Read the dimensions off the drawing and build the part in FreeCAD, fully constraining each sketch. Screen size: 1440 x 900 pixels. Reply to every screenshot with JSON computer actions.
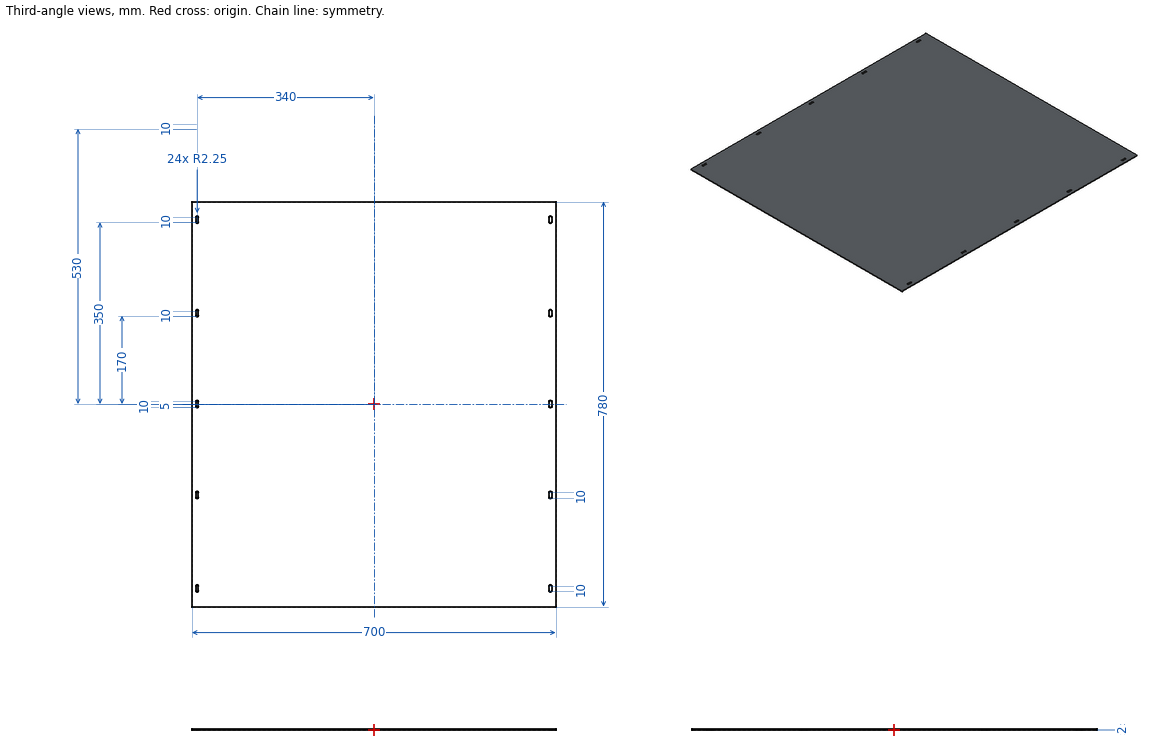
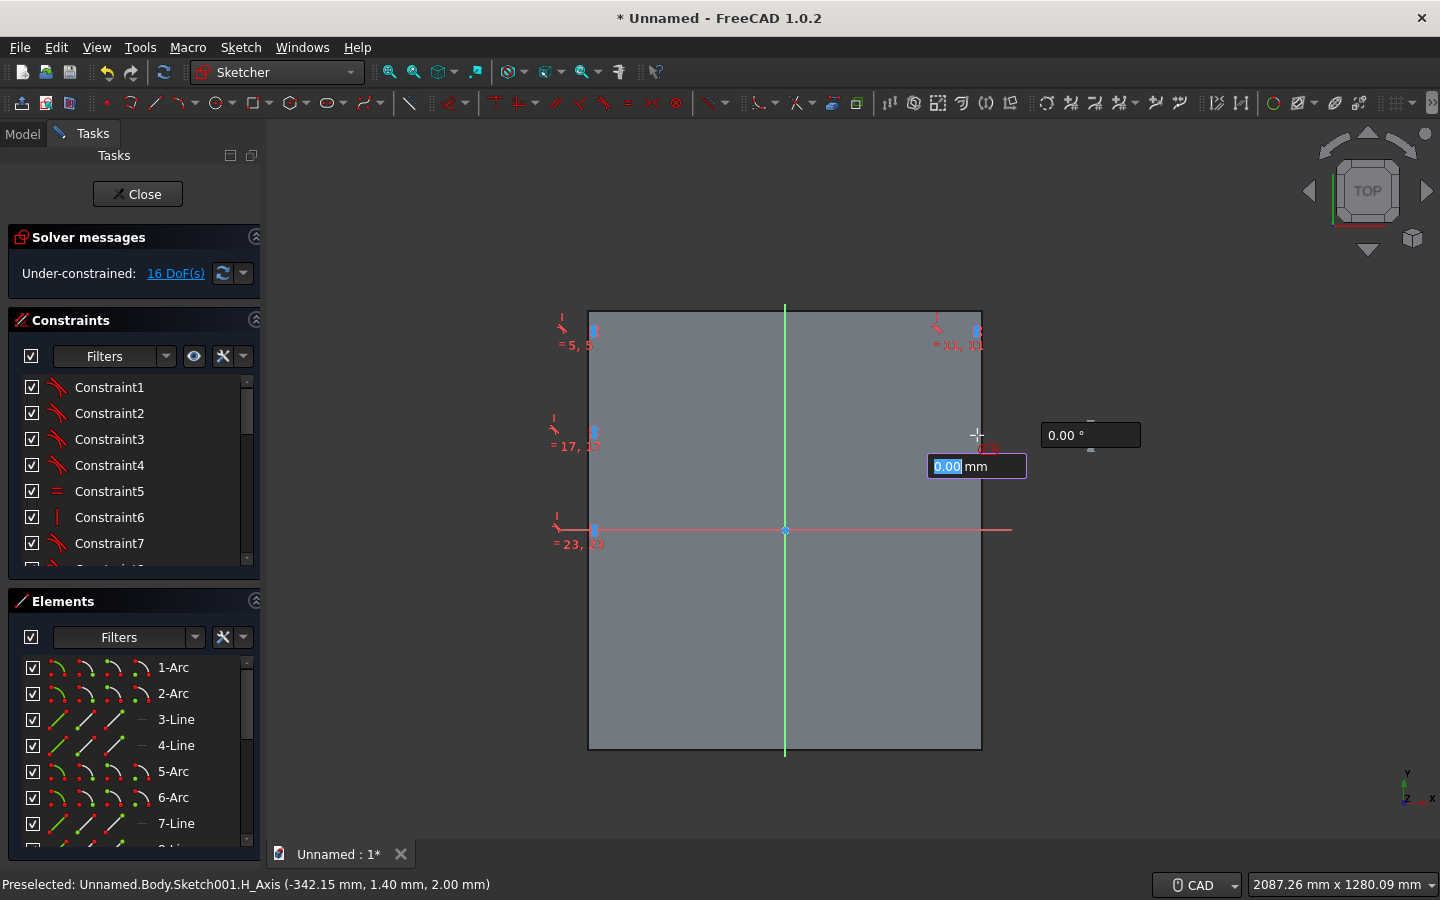
{"action": "scroll", "coordinate": [977, 429], "scroll_direction": "up", "scroll_amount": 6}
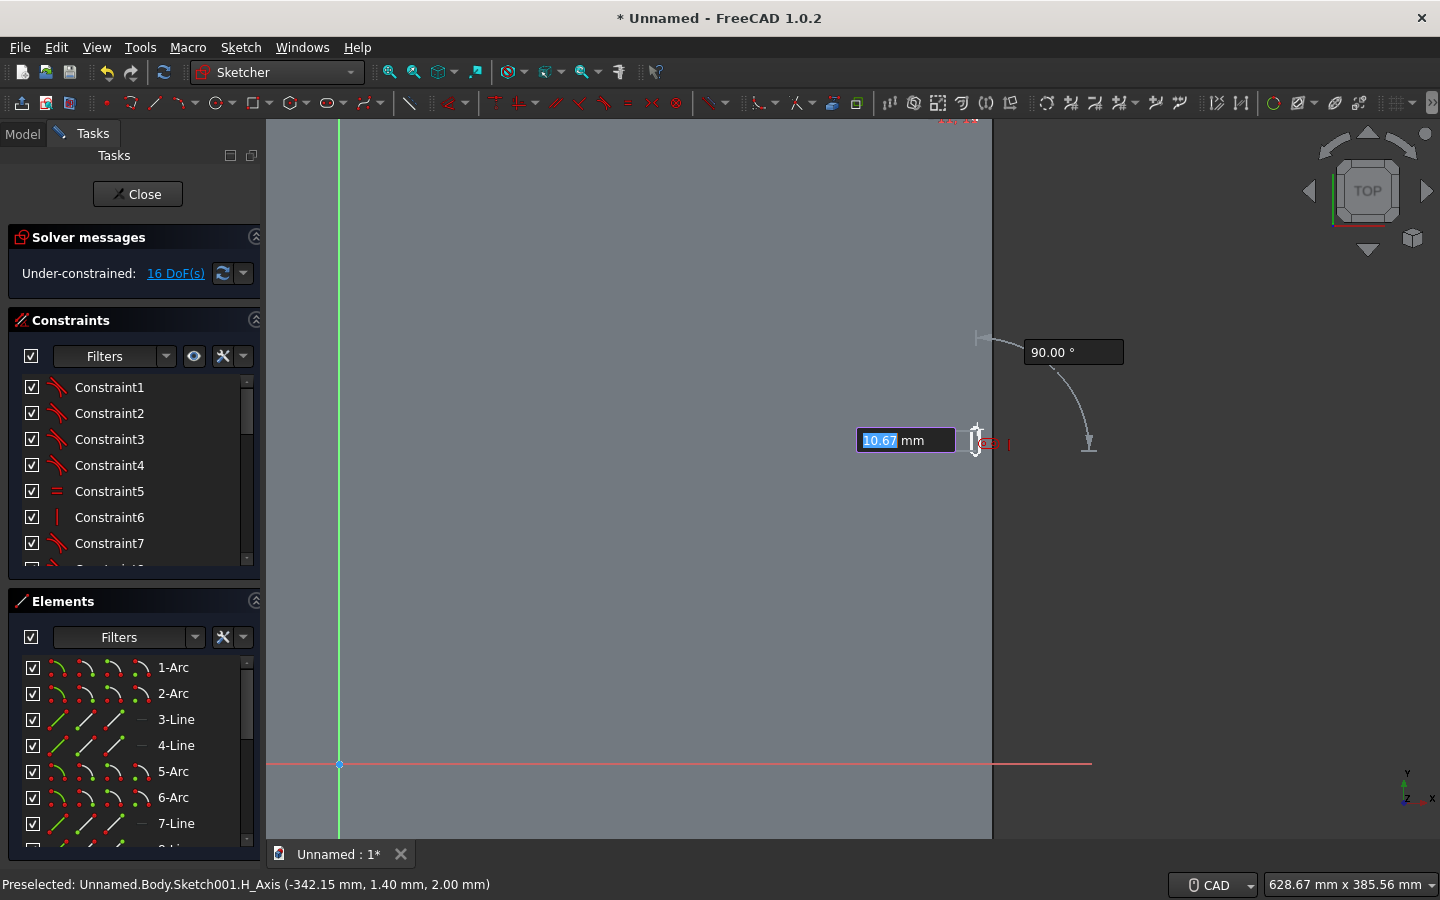
{"action": "left_click", "coordinate": [976, 428]}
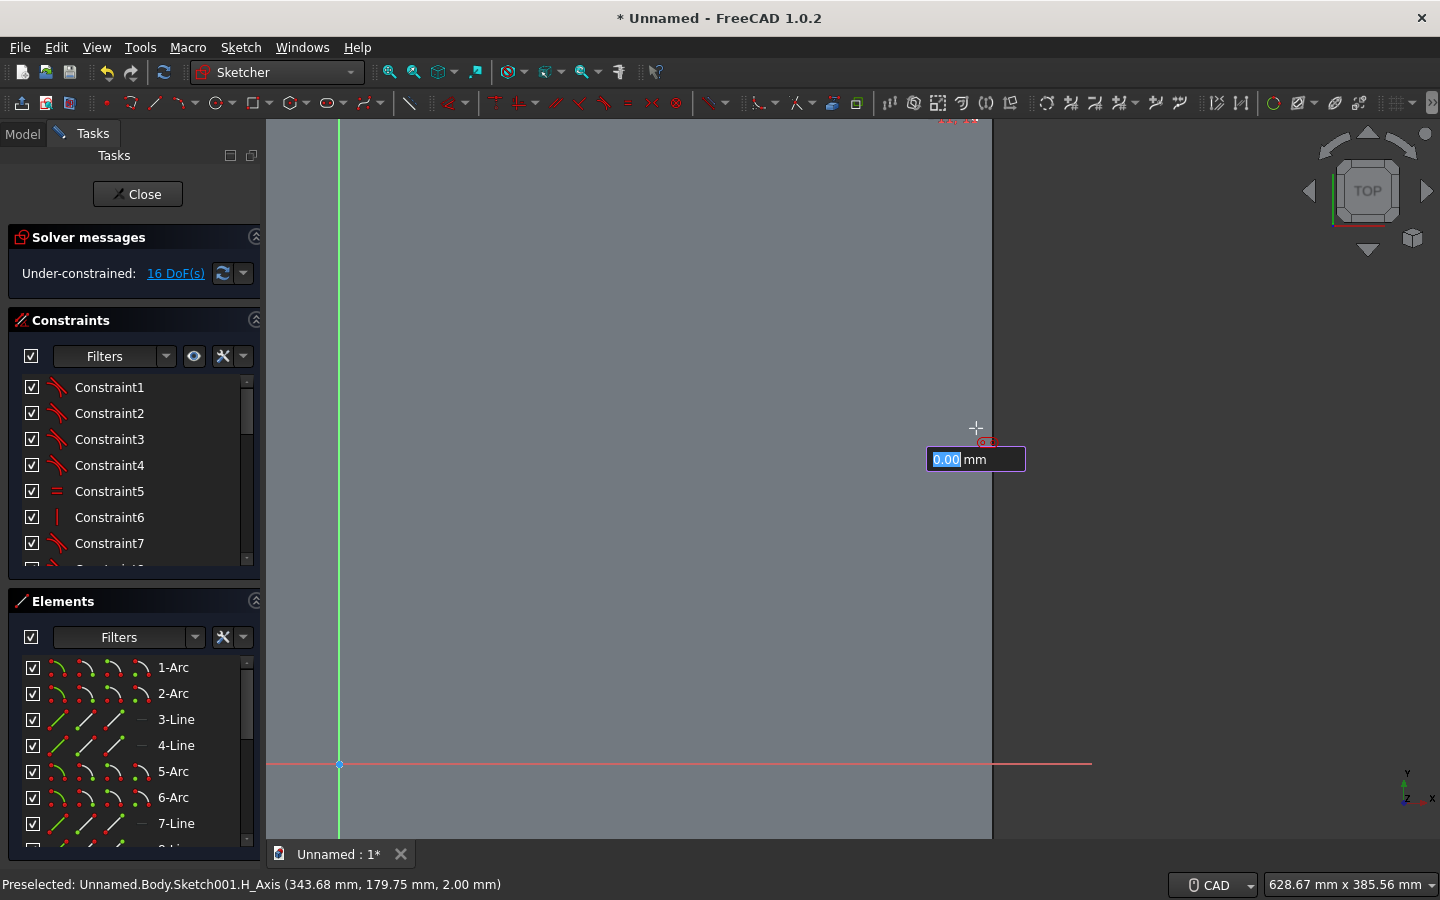
{"action": "scroll", "coordinate": [978, 437], "scroll_direction": "up", "scroll_amount": 7}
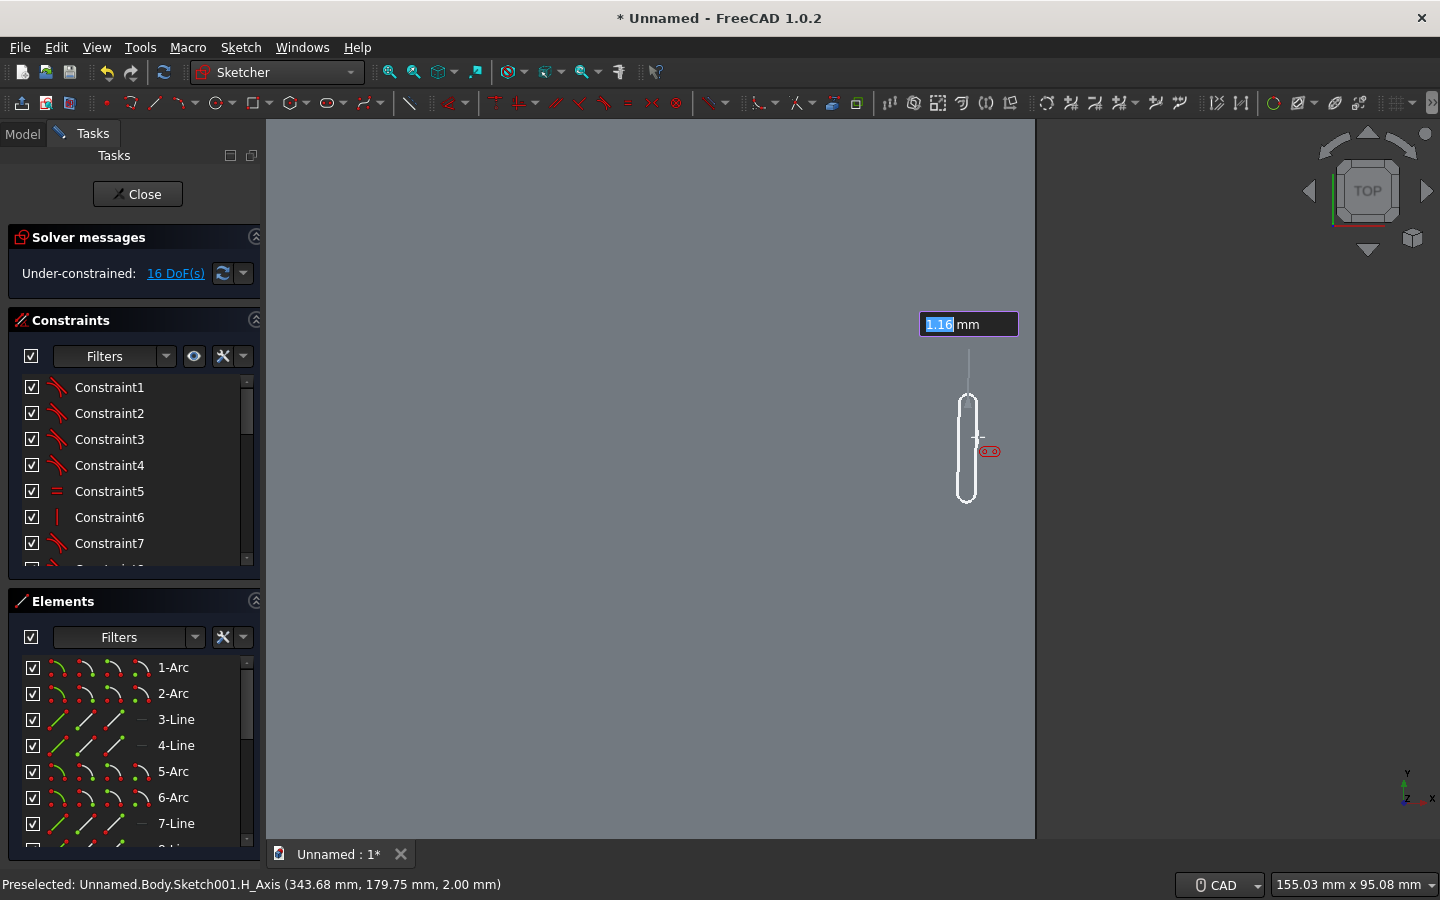
{"action": "left_click", "coordinate": [977, 437]}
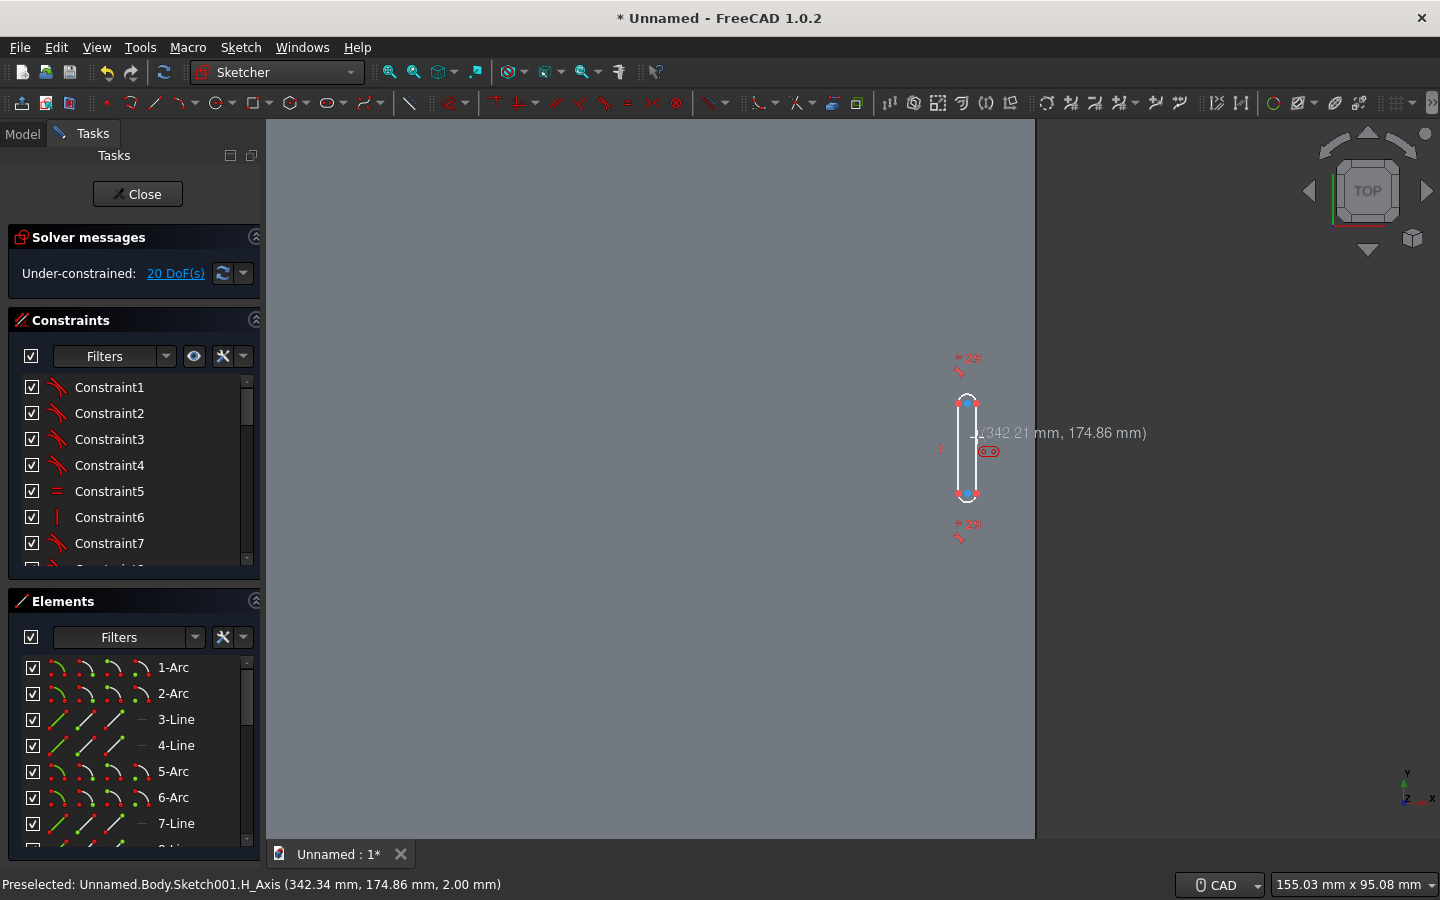
{"action": "scroll", "coordinate": [977, 431], "scroll_direction": "down", "scroll_amount": 13}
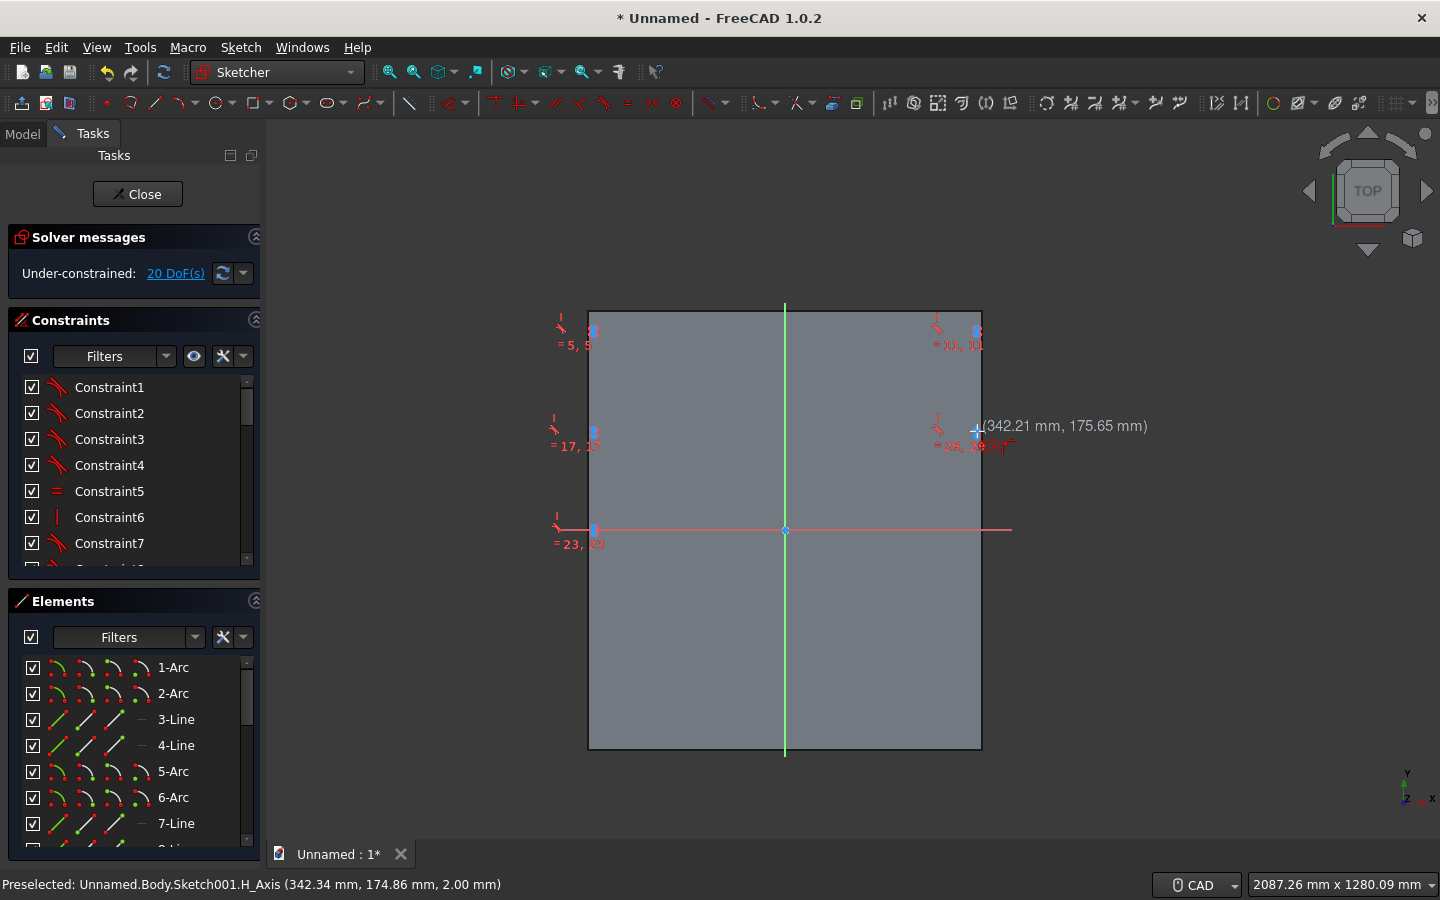
{"action": "scroll", "coordinate": [976, 533], "scroll_direction": "up", "scroll_amount": 15}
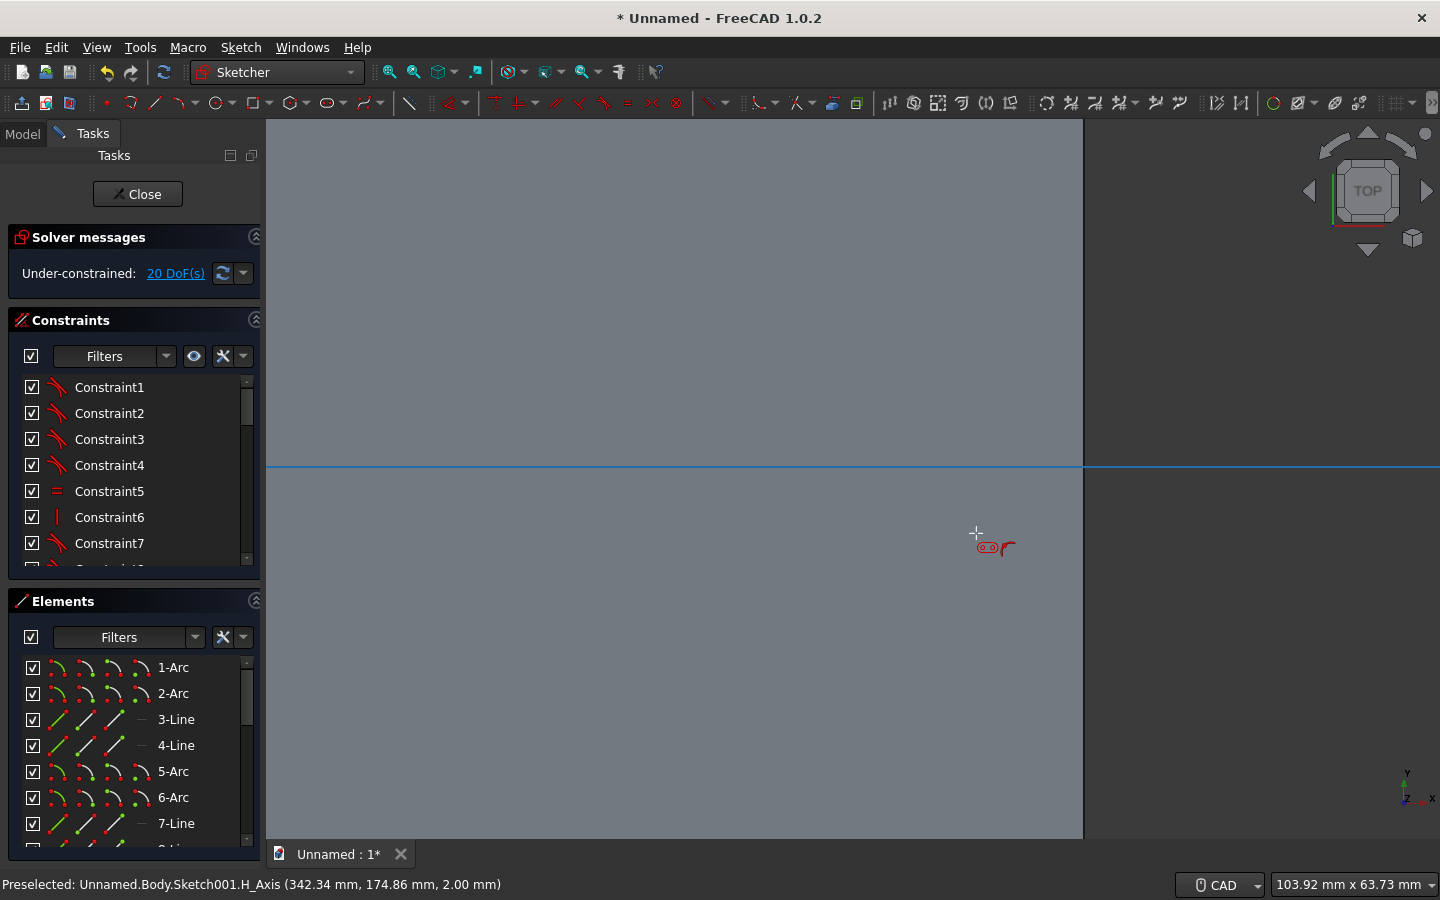
{"action": "scroll", "coordinate": [976, 533], "scroll_direction": "down", "scroll_amount": 15}